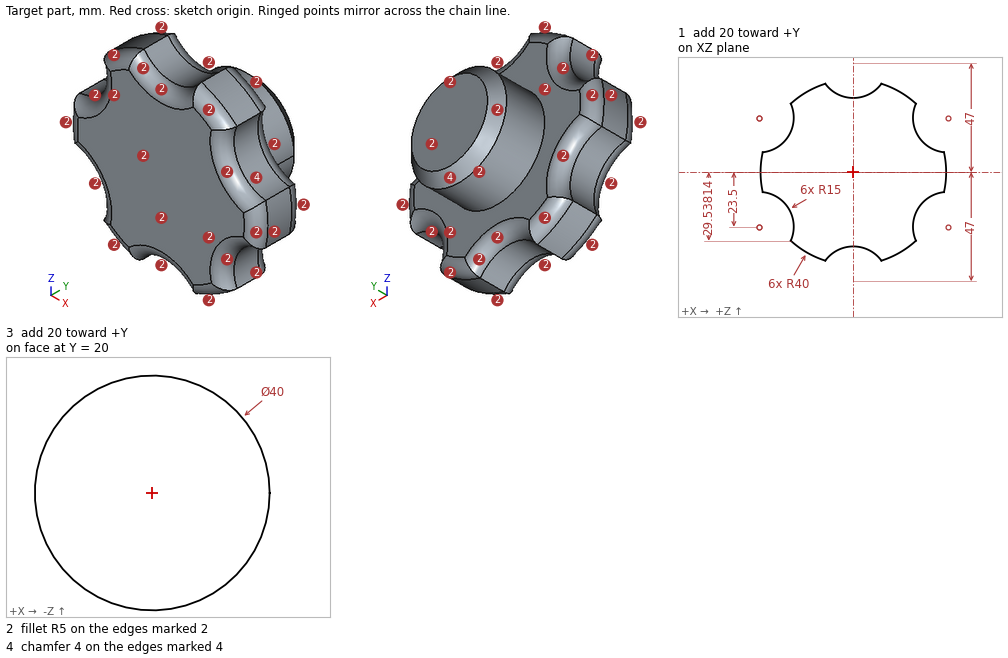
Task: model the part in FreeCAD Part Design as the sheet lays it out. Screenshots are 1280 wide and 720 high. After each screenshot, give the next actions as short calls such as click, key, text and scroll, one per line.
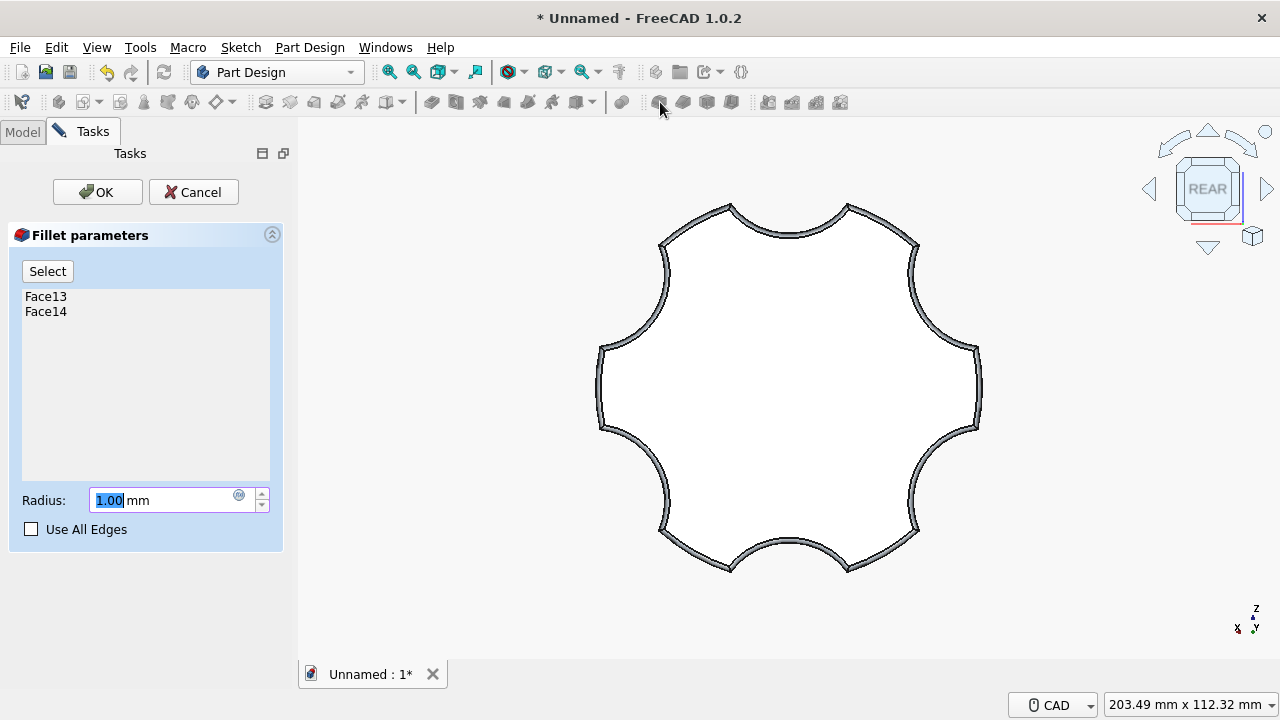
text(5)
key(Tab)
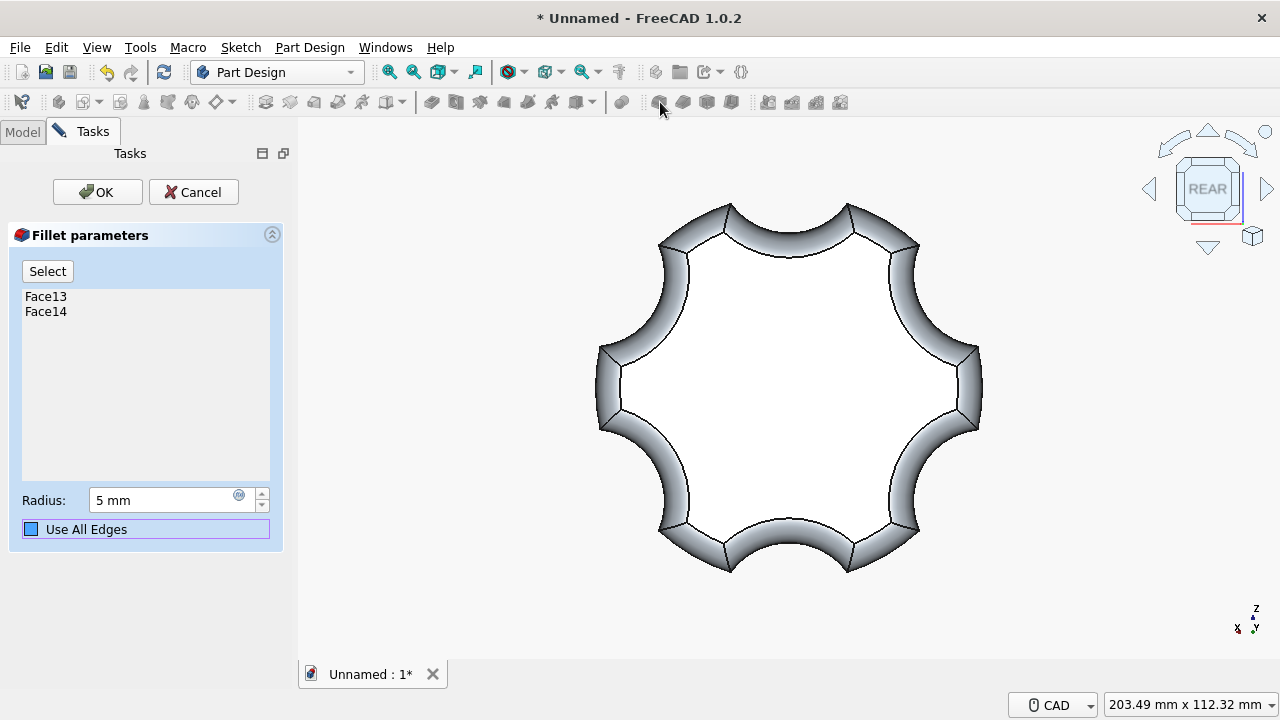
click(98, 192)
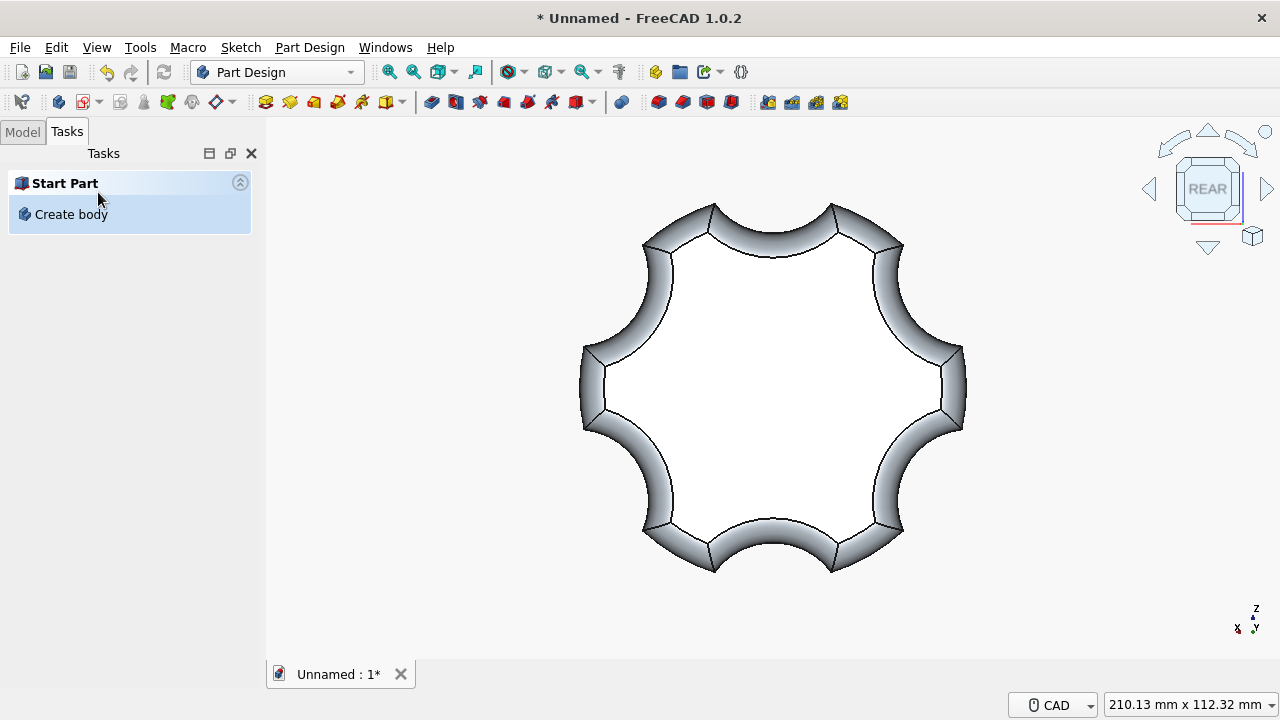
click(773, 387)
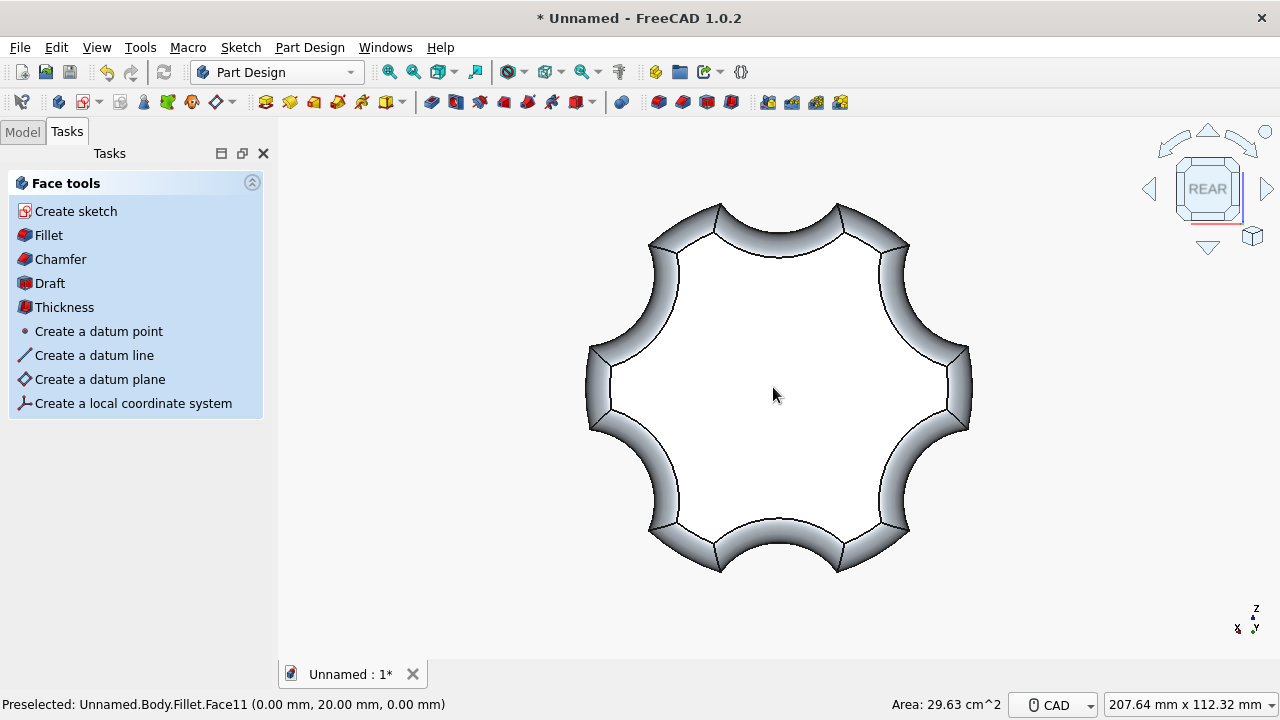
click(84, 102)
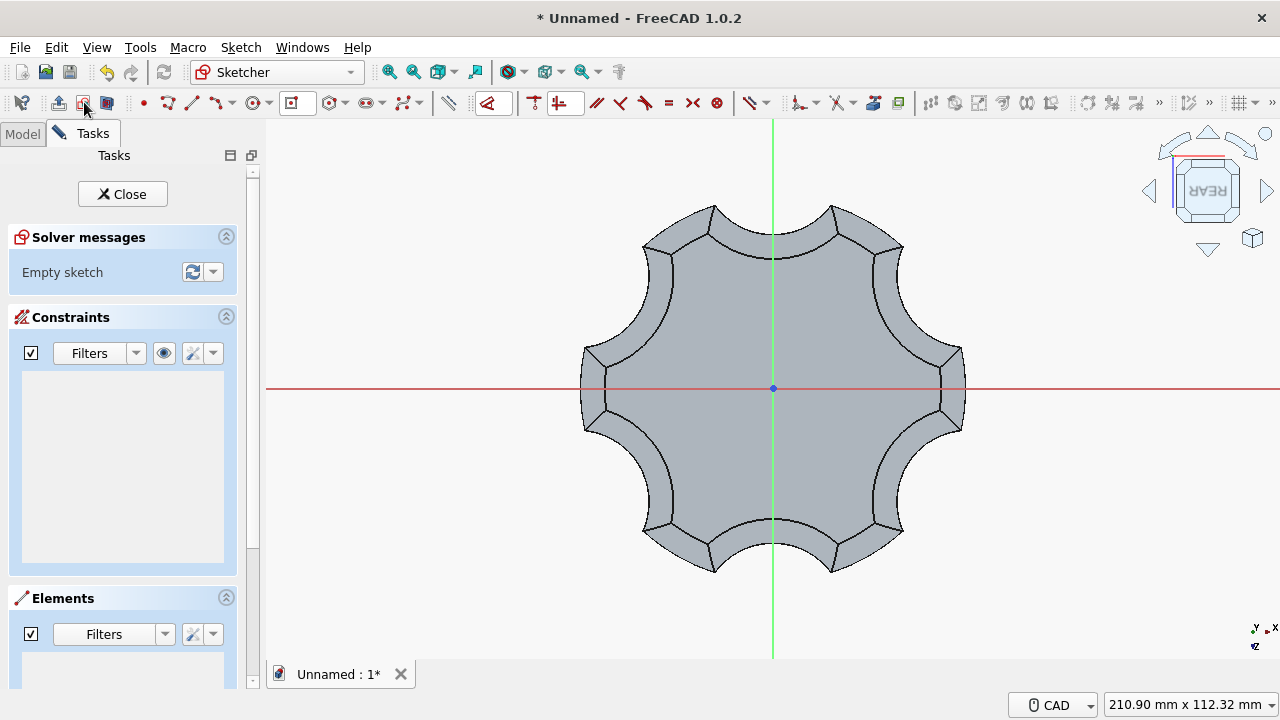
scroll(856, 389, up, 3)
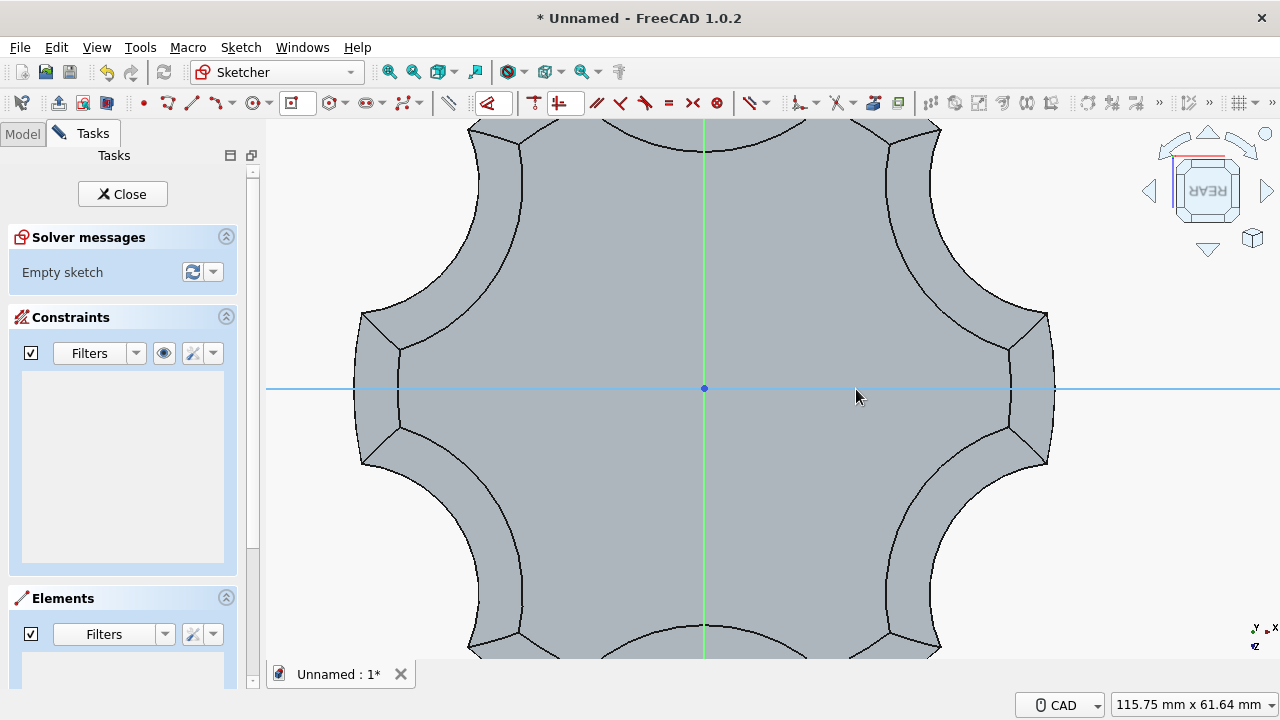
click(254, 104)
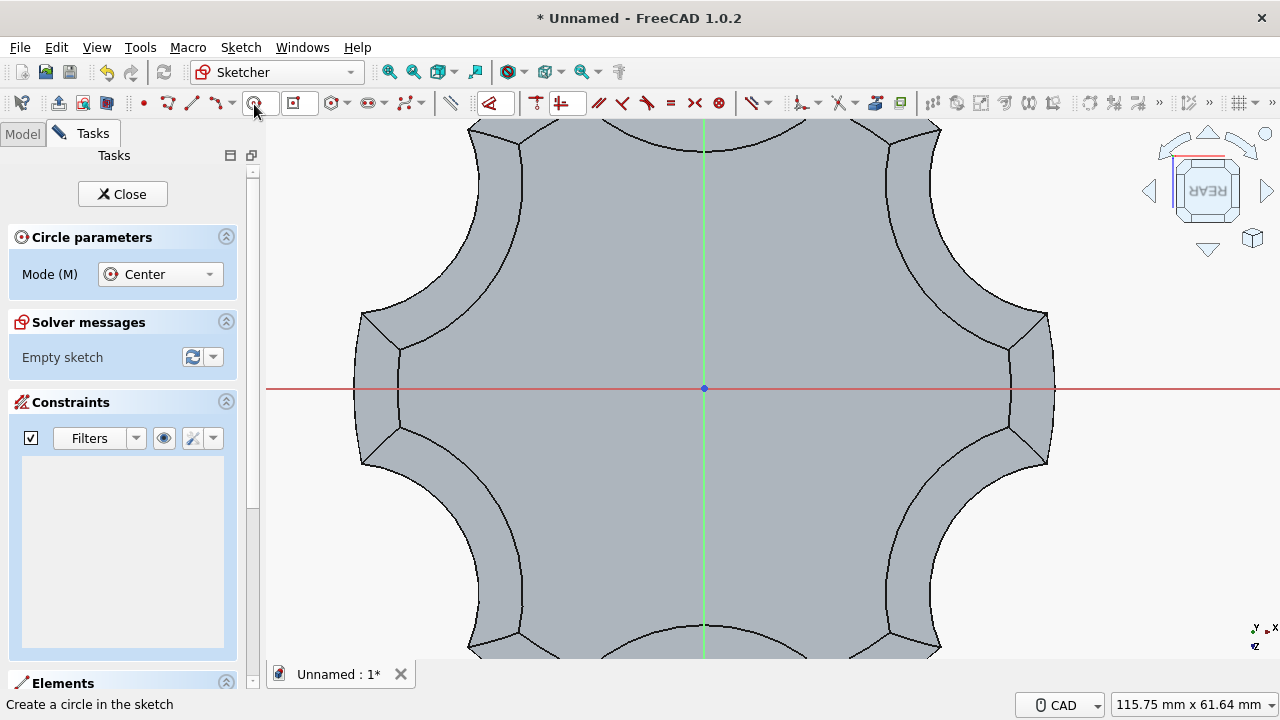
click(704, 389)
click(828, 265)
key(Escape)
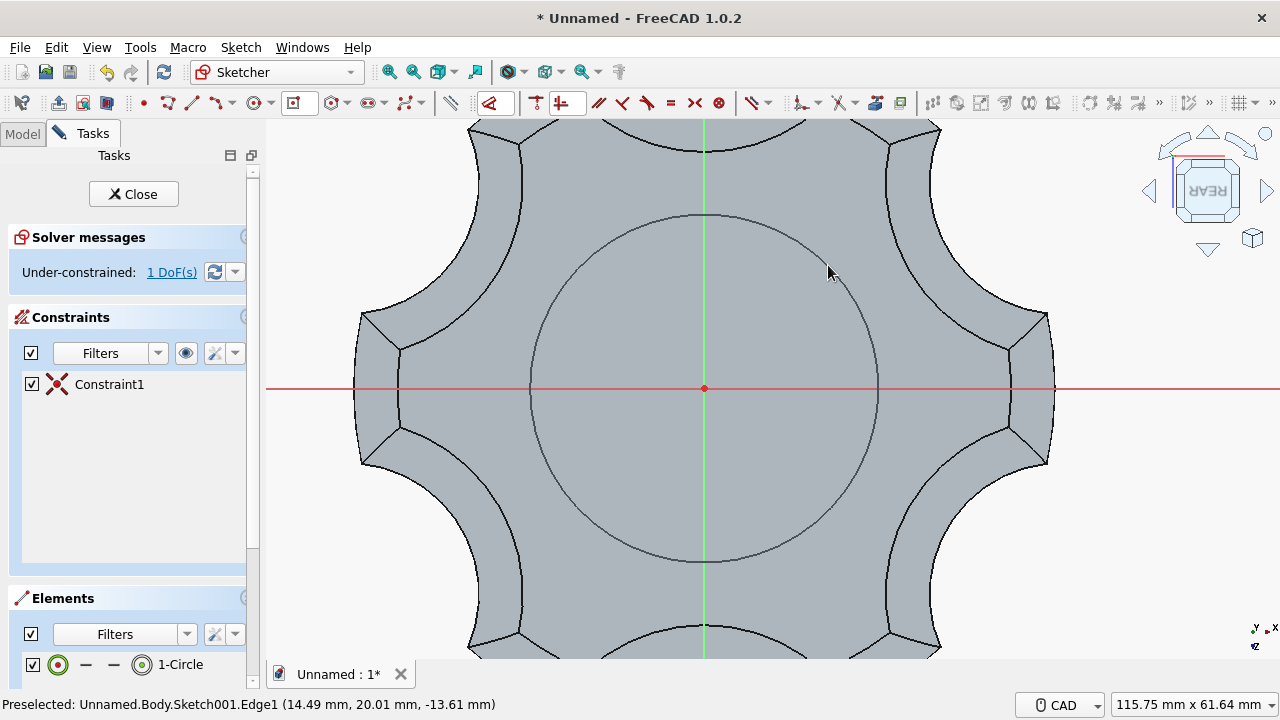
click(827, 265)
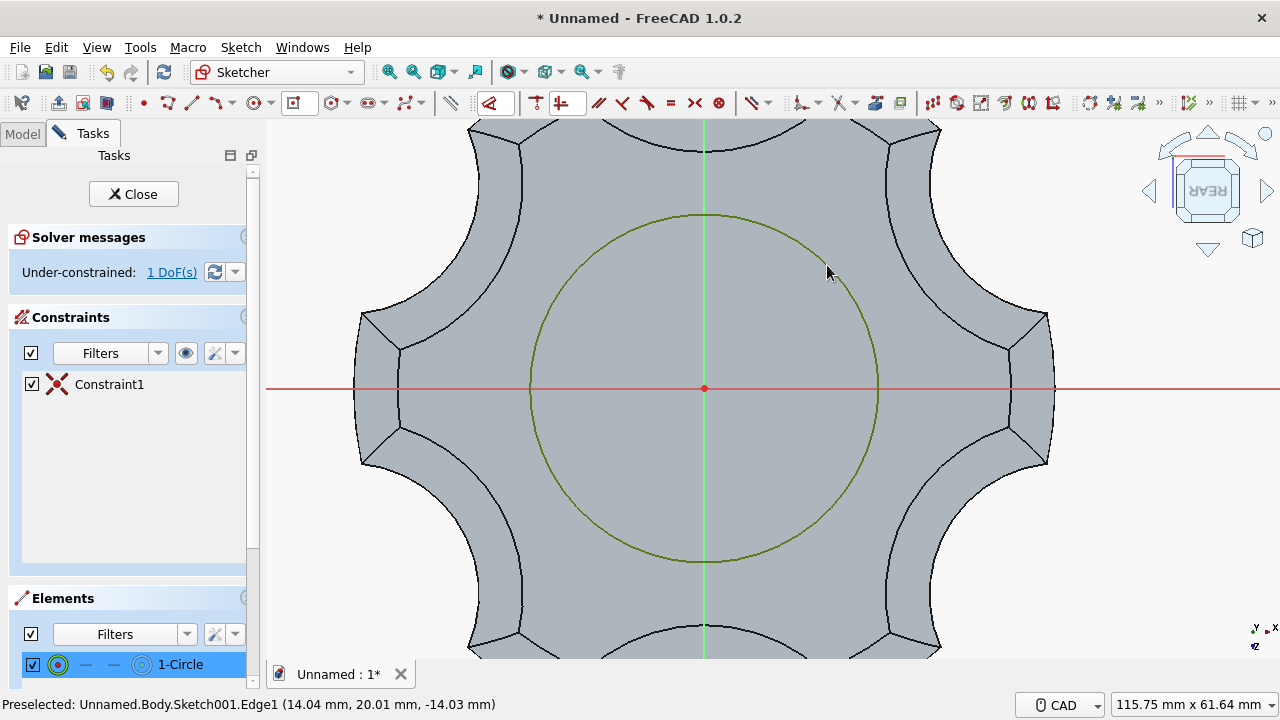
click(508, 104)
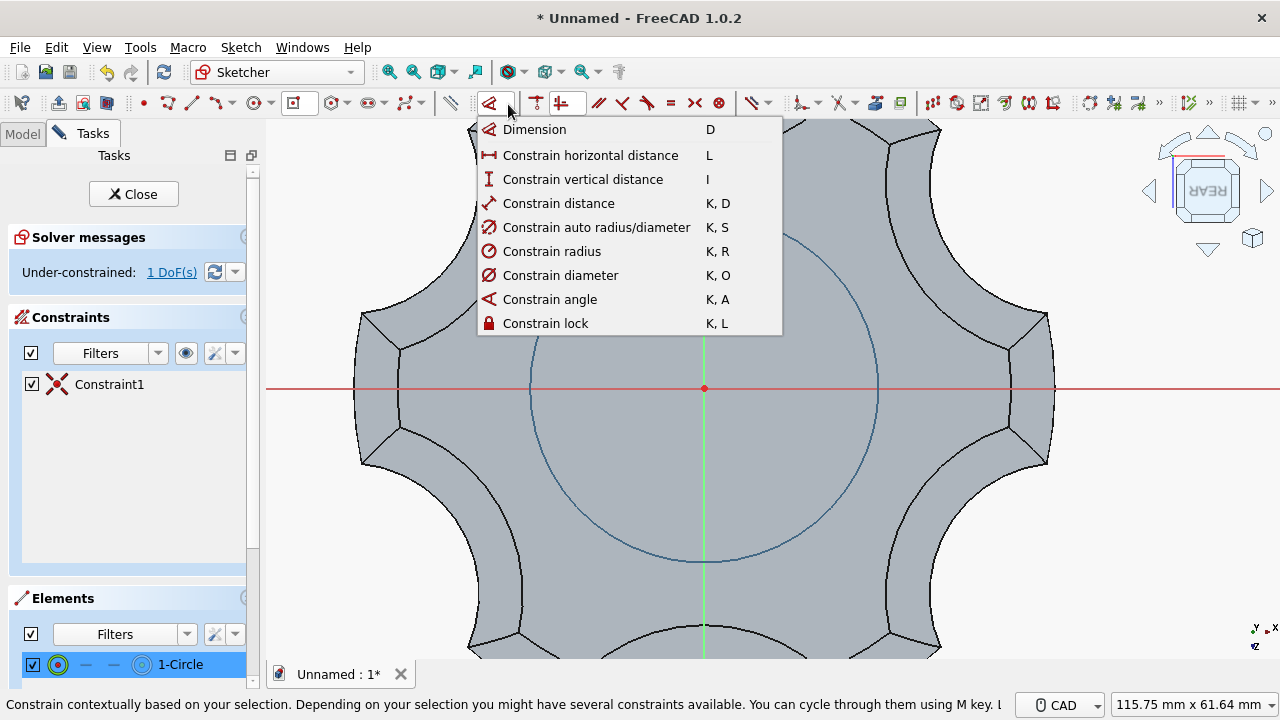
click(630, 275)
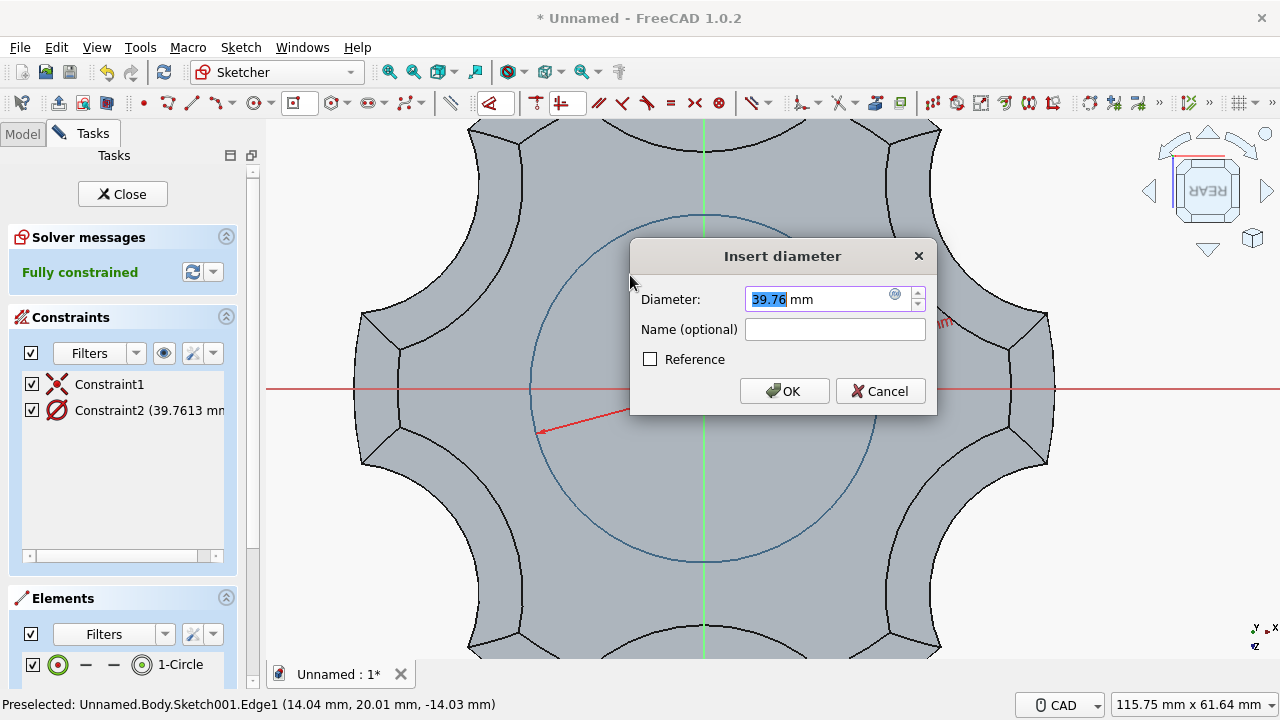
text(40)
key(Return)